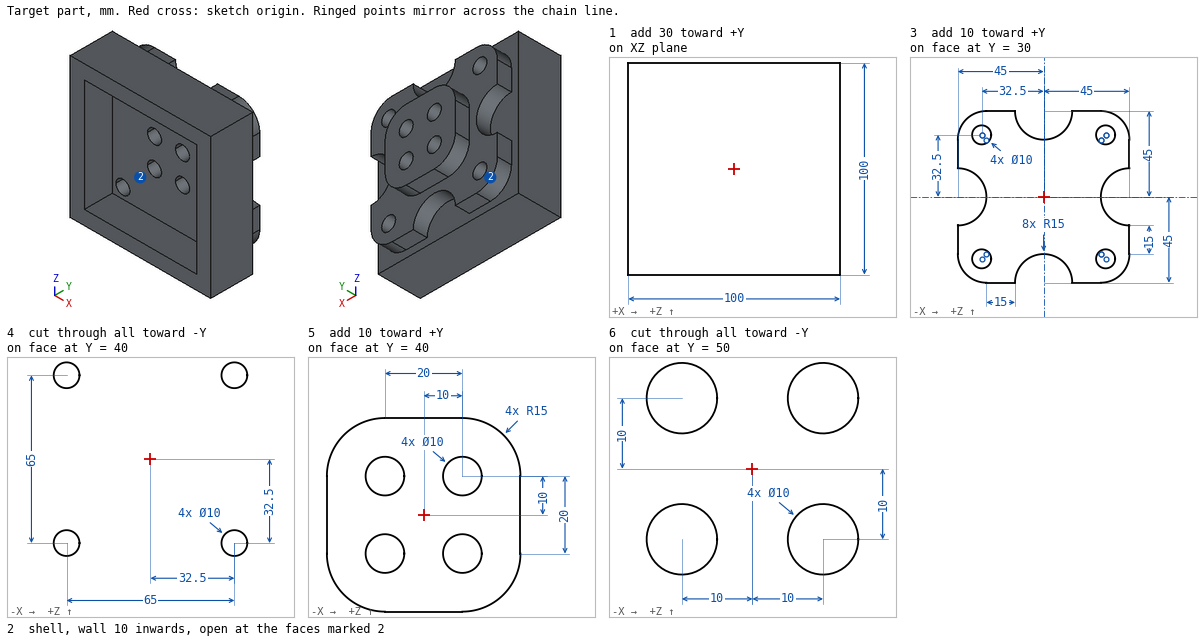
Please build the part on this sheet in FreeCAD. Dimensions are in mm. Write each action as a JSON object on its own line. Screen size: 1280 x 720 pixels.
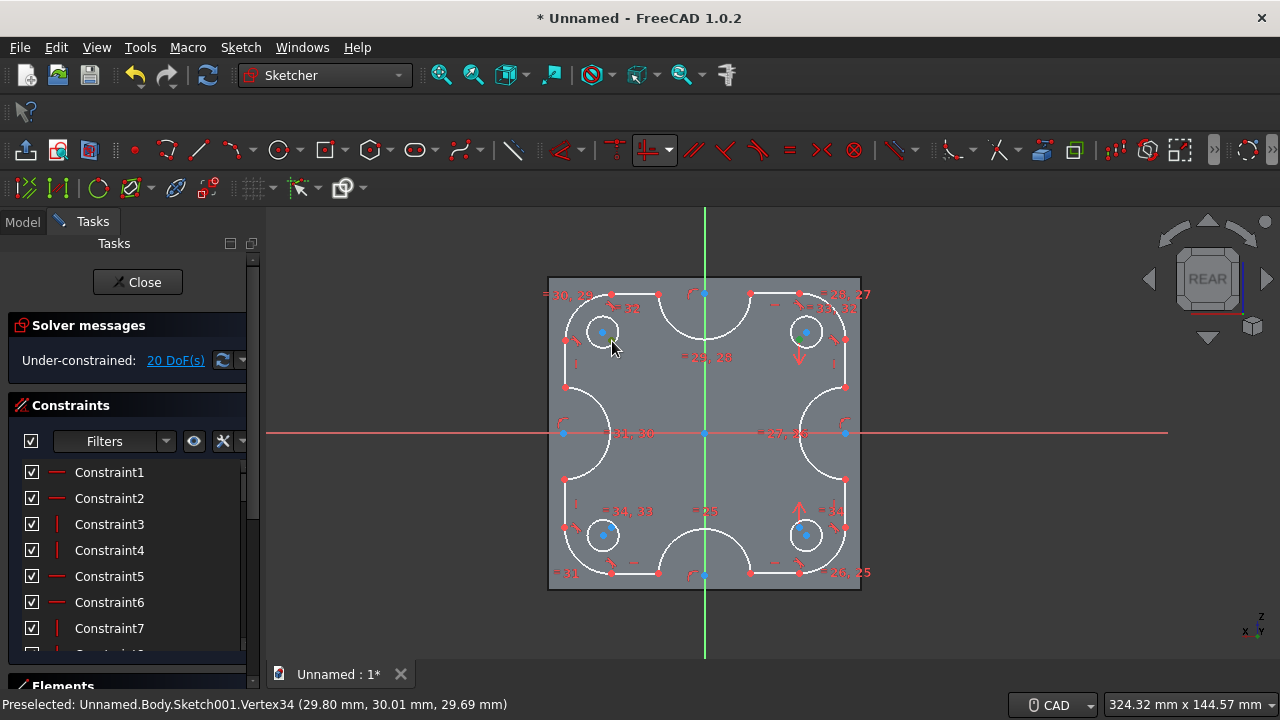
{"action": "left_click", "coordinate": [705, 603]}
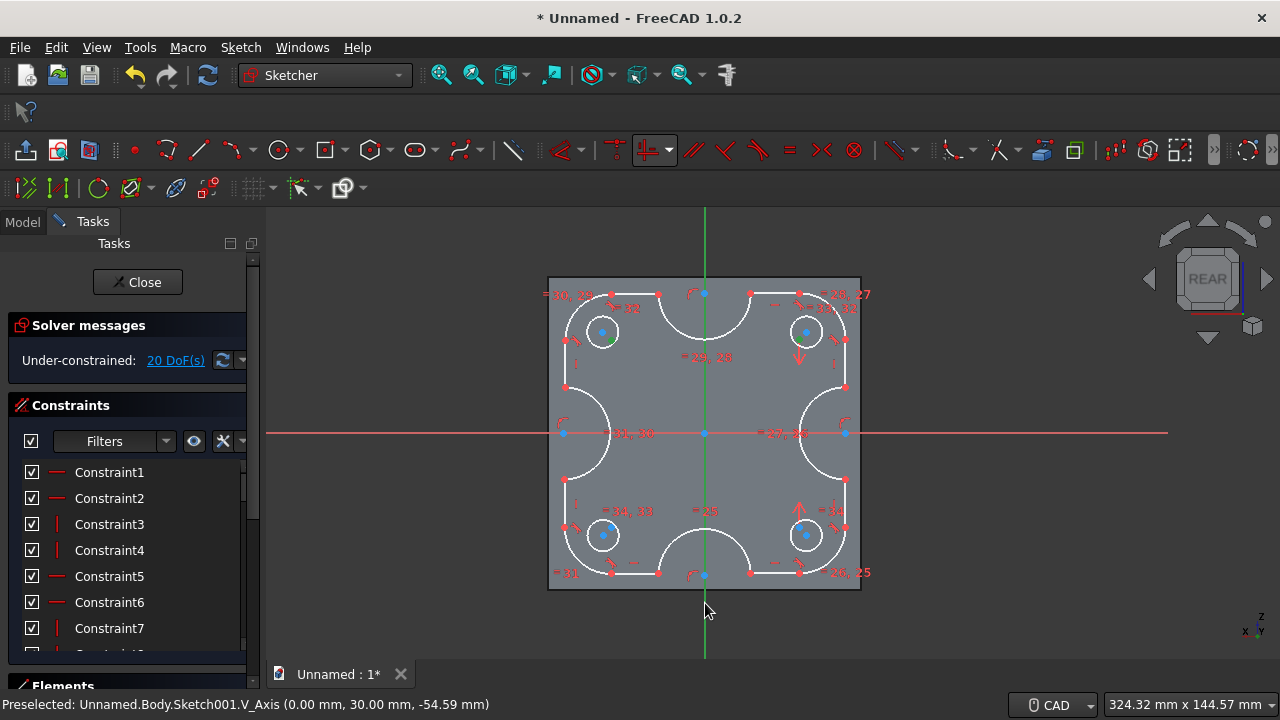
{"action": "left_click", "coordinate": [822, 150]}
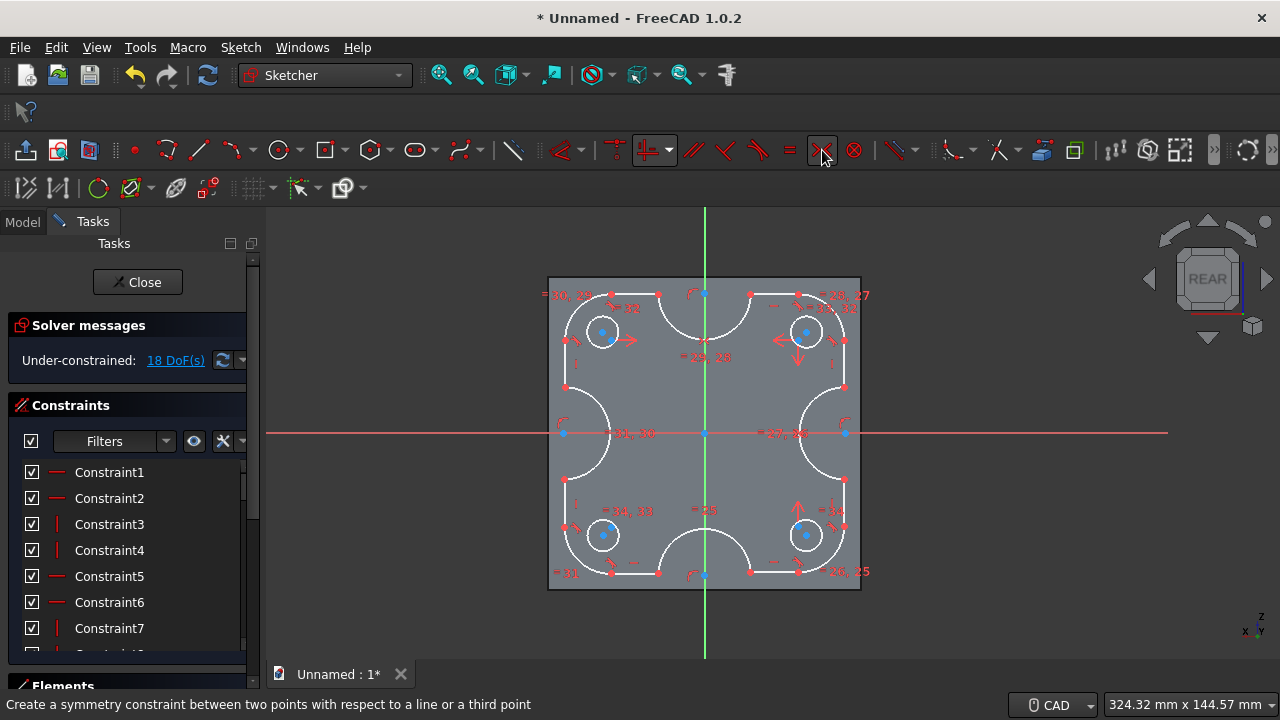
{"action": "left_click", "coordinate": [798, 526]}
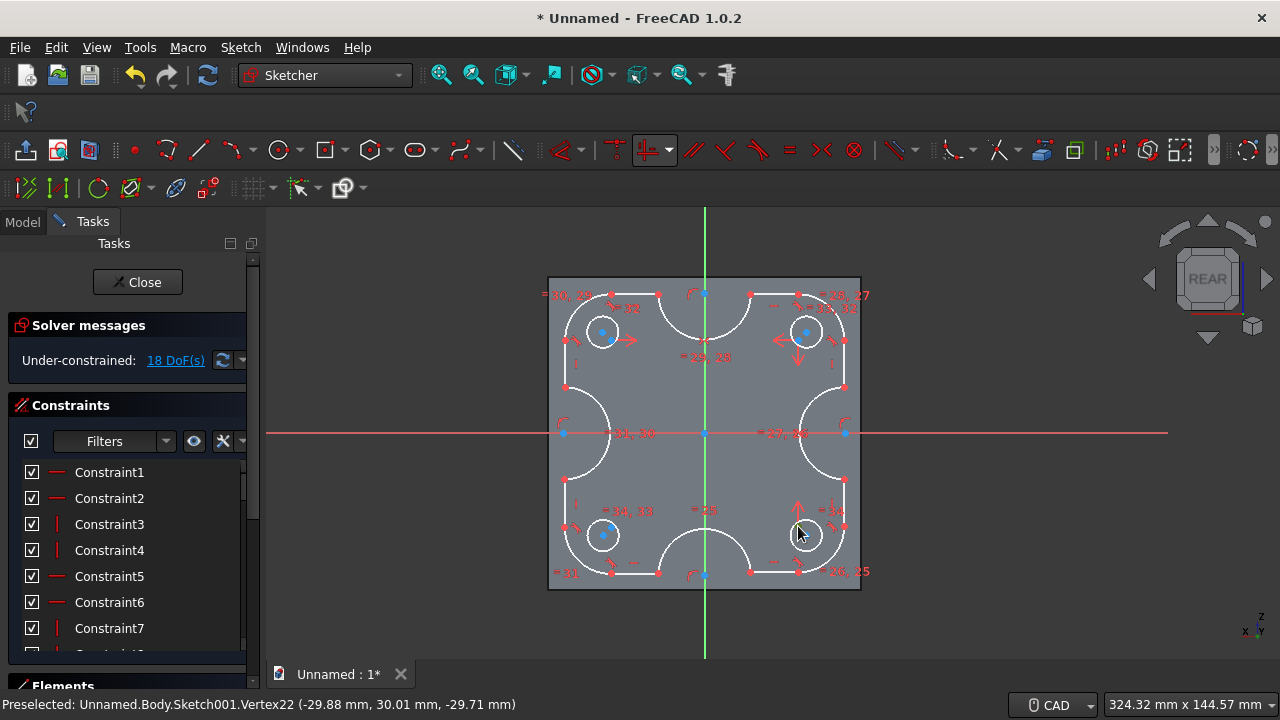
{"action": "left_click", "coordinate": [611, 528]}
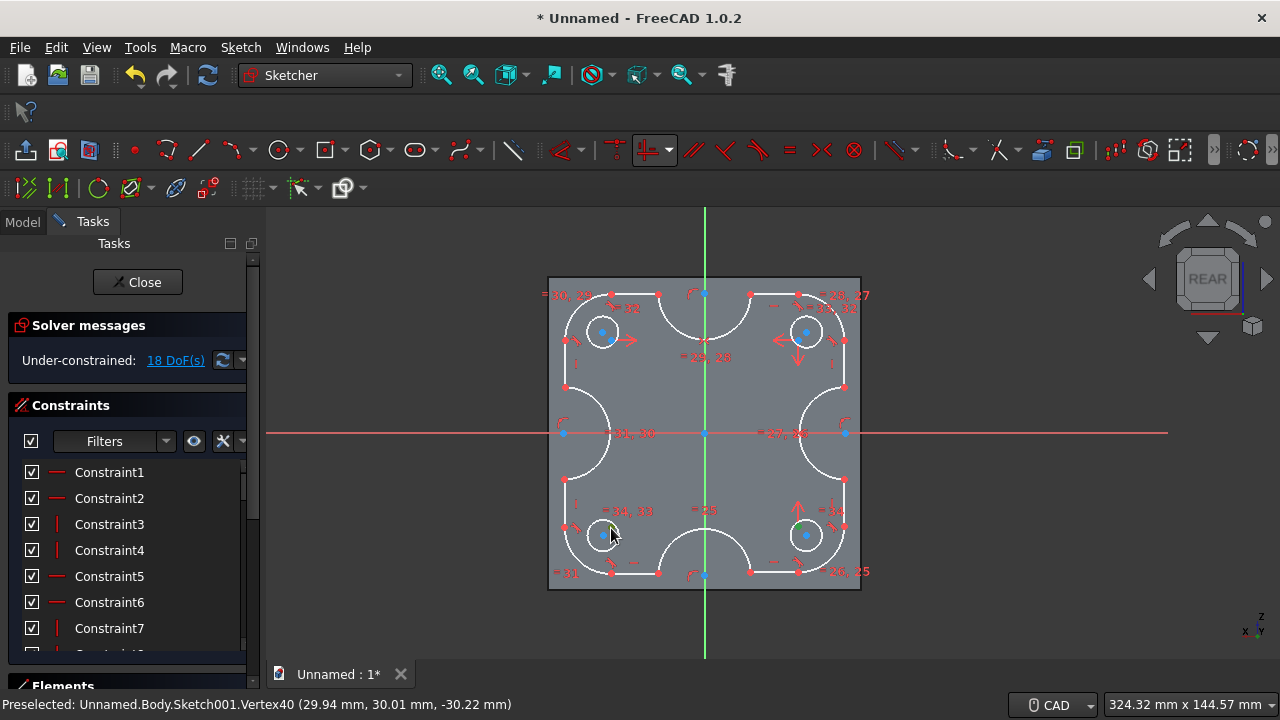
{"action": "left_click", "coordinate": [705, 603]}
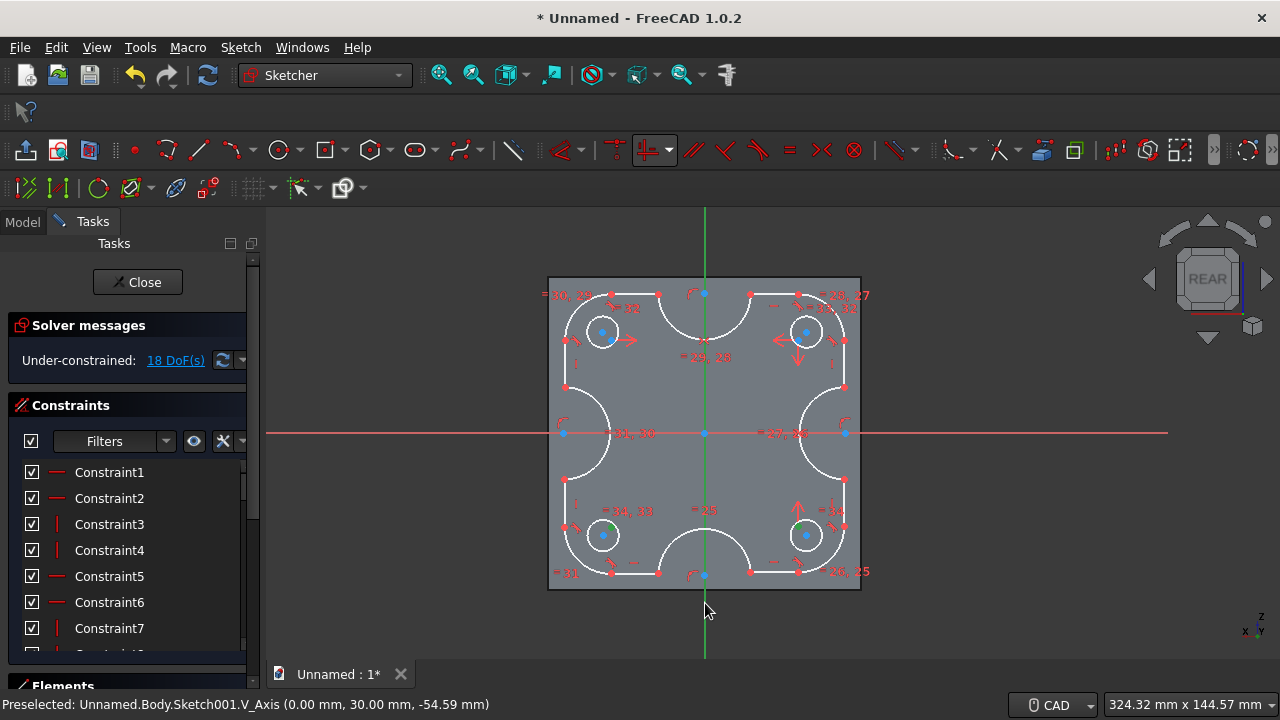
{"action": "left_click", "coordinate": [822, 150]}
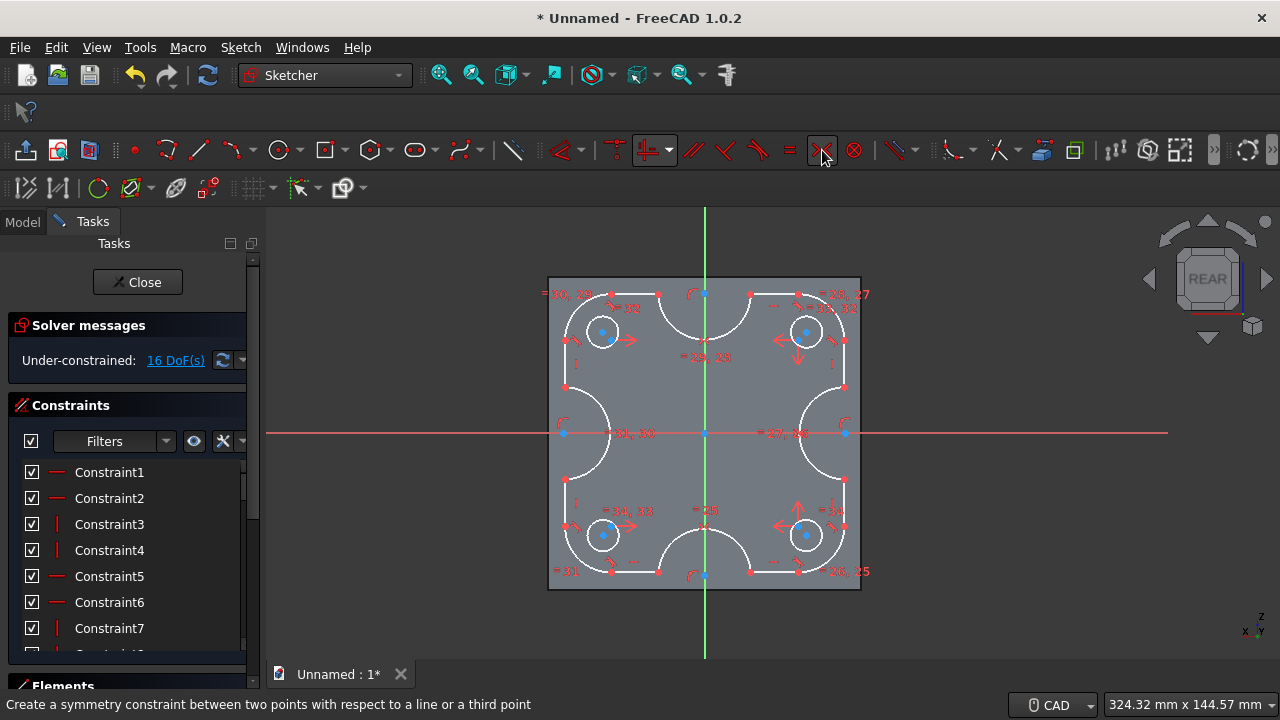
{"action": "left_click", "coordinate": [603, 332]}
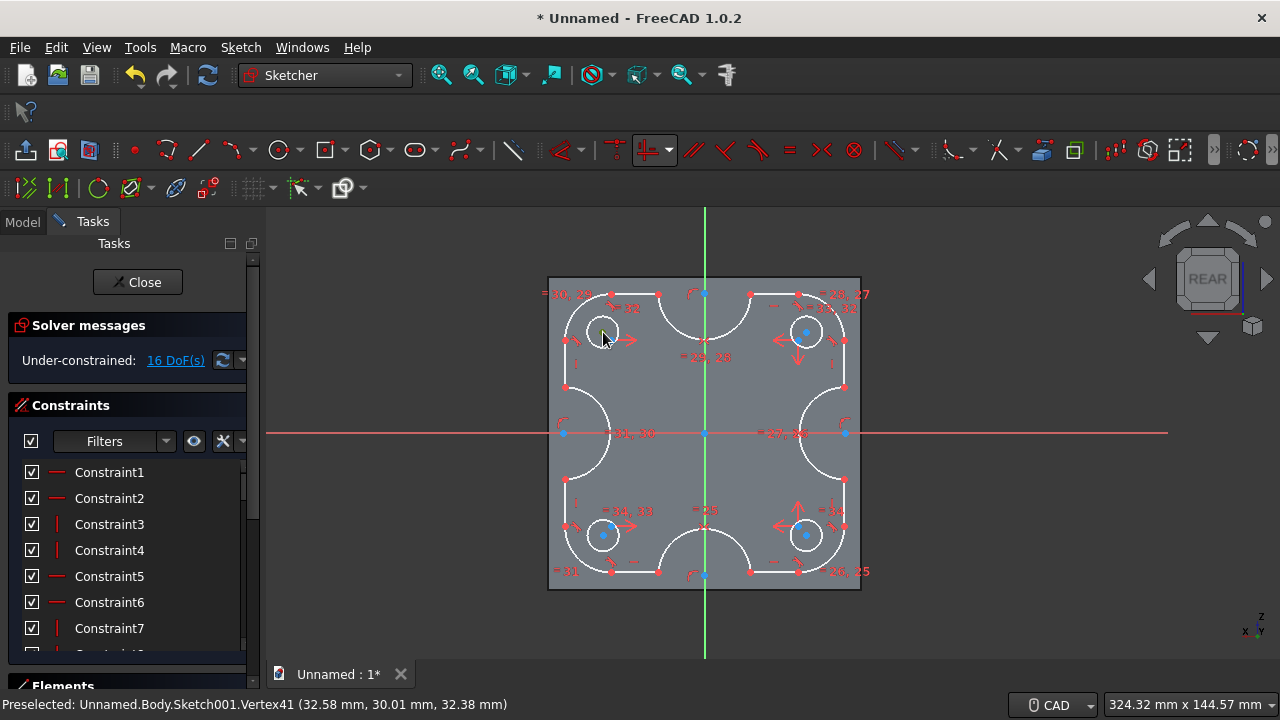
{"action": "left_click", "coordinate": [807, 332]}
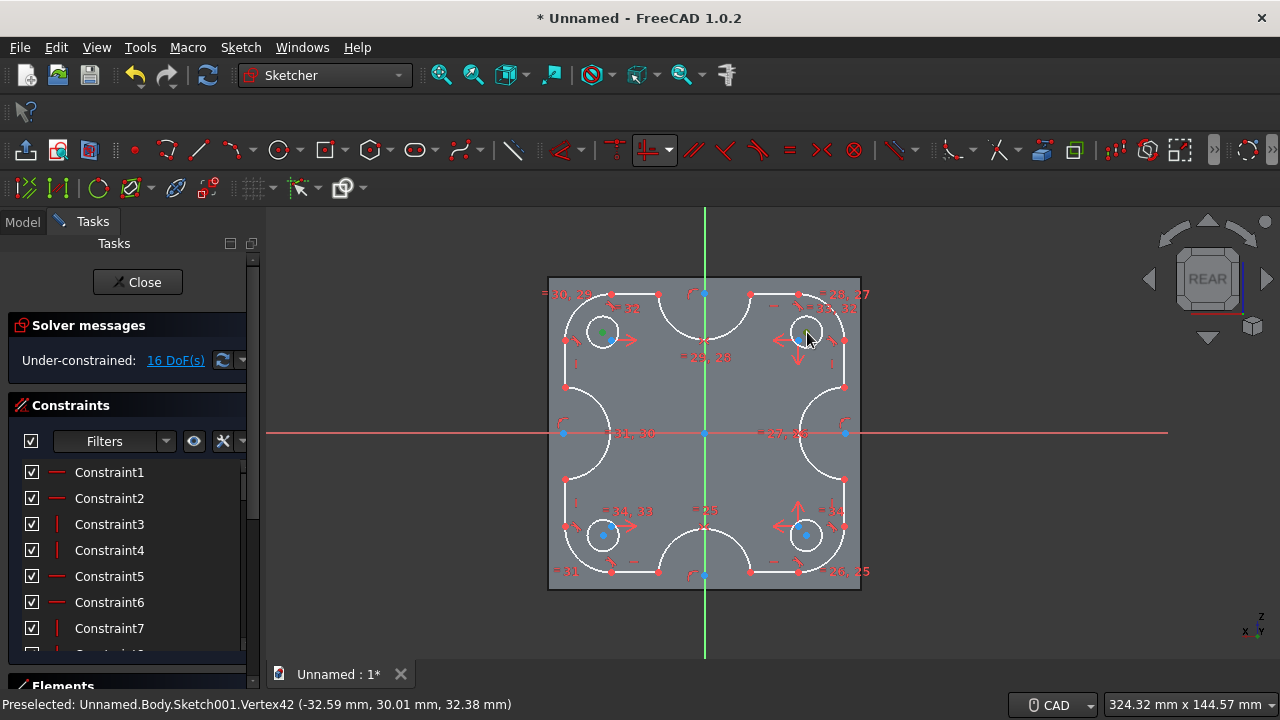
{"action": "left_click", "coordinate": [705, 603]}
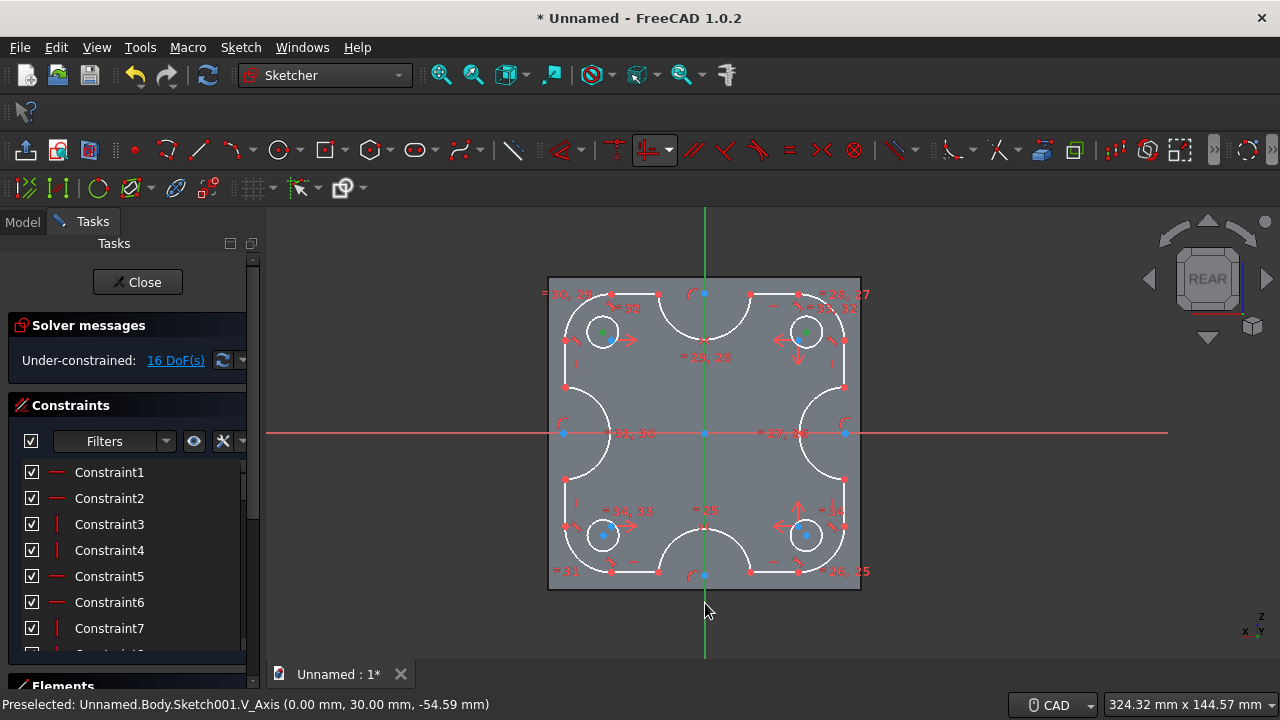
{"action": "left_click", "coordinate": [822, 150]}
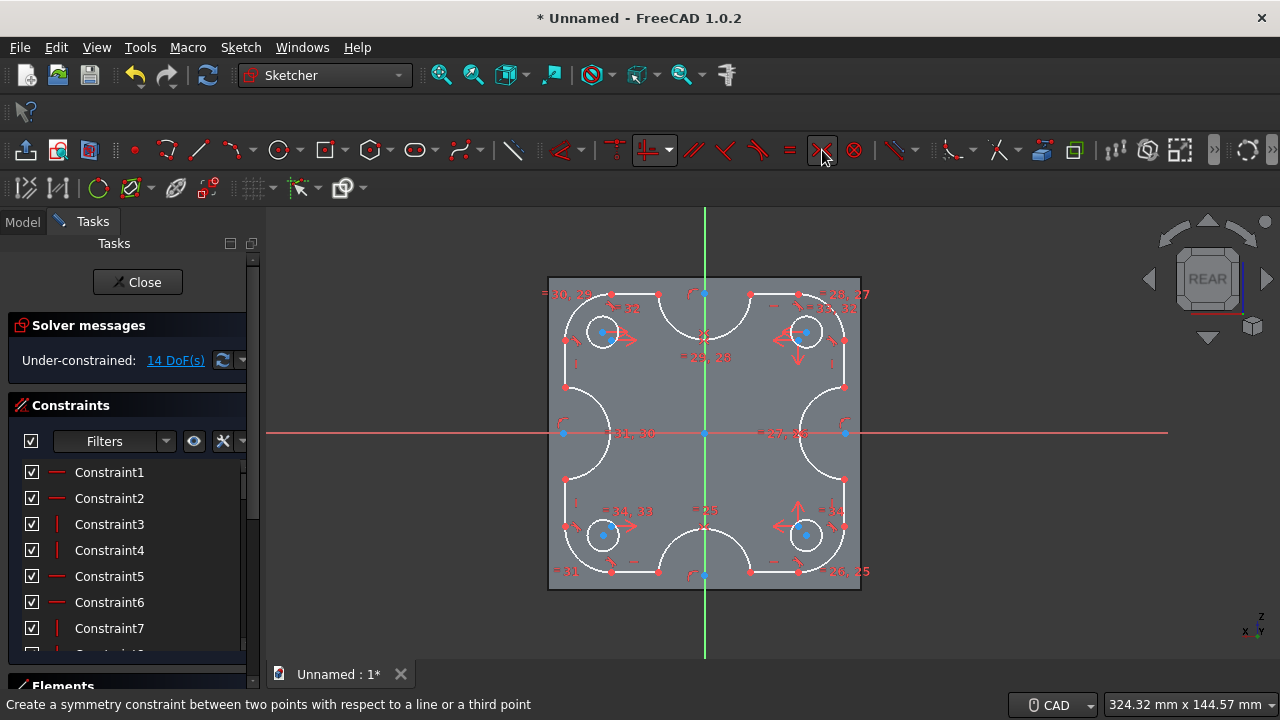
{"action": "left_click", "coordinate": [603, 332]}